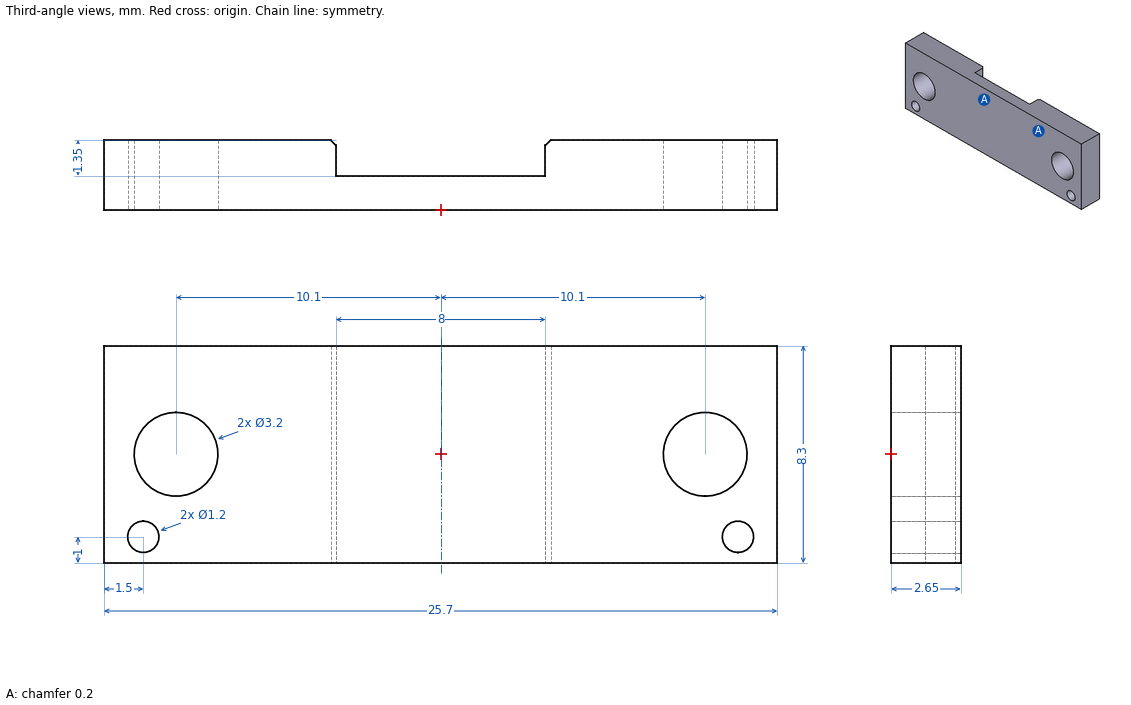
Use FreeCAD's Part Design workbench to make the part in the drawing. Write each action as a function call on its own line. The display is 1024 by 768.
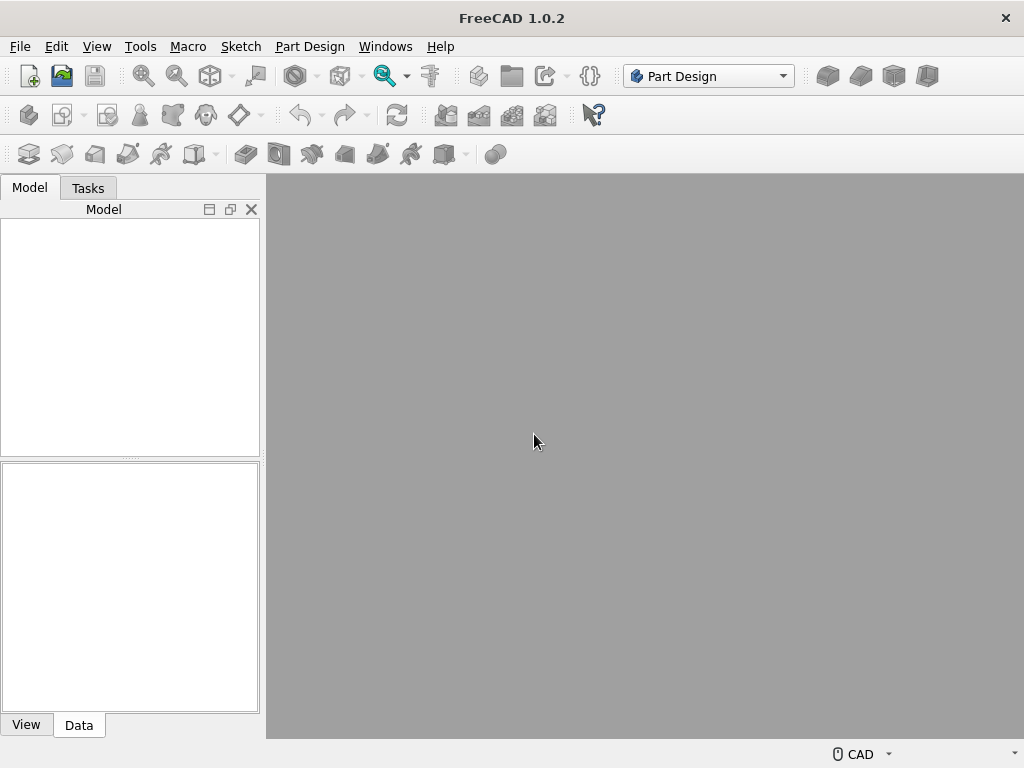
click(29, 76)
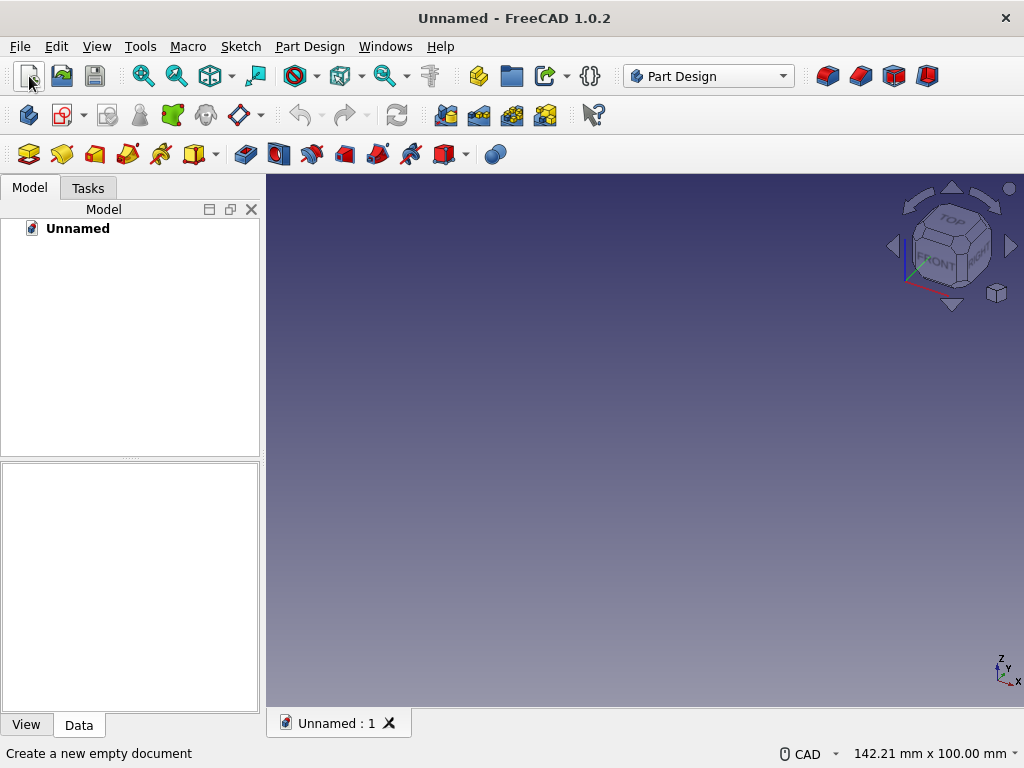
click(62, 116)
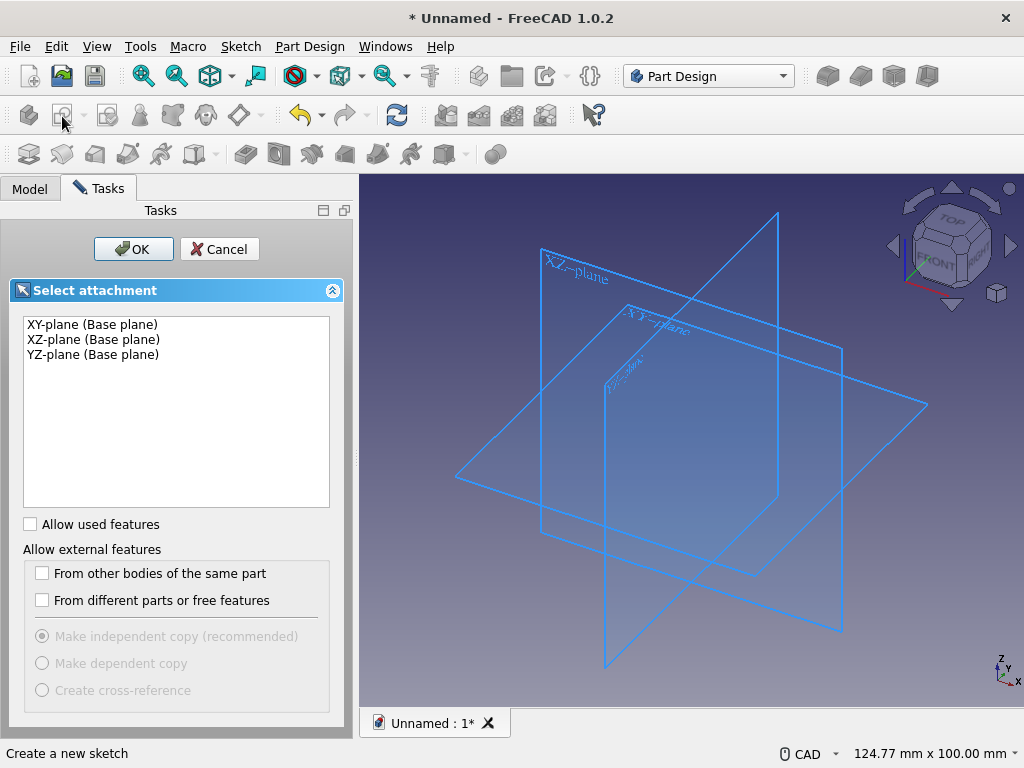
click(84, 340)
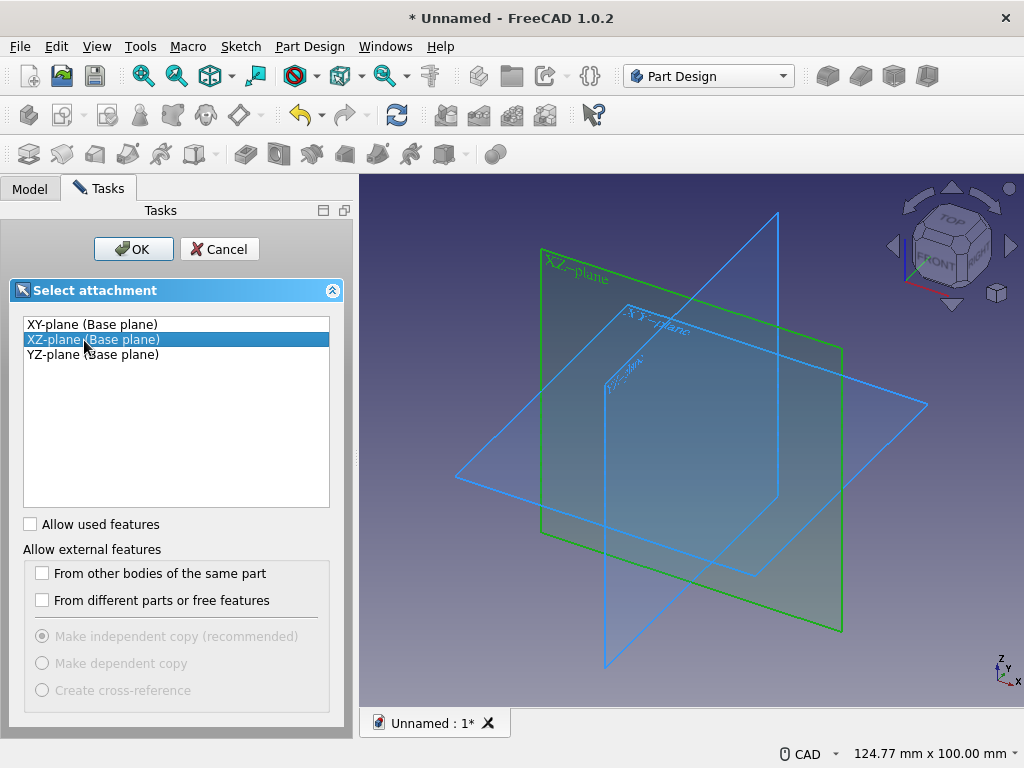
click(134, 249)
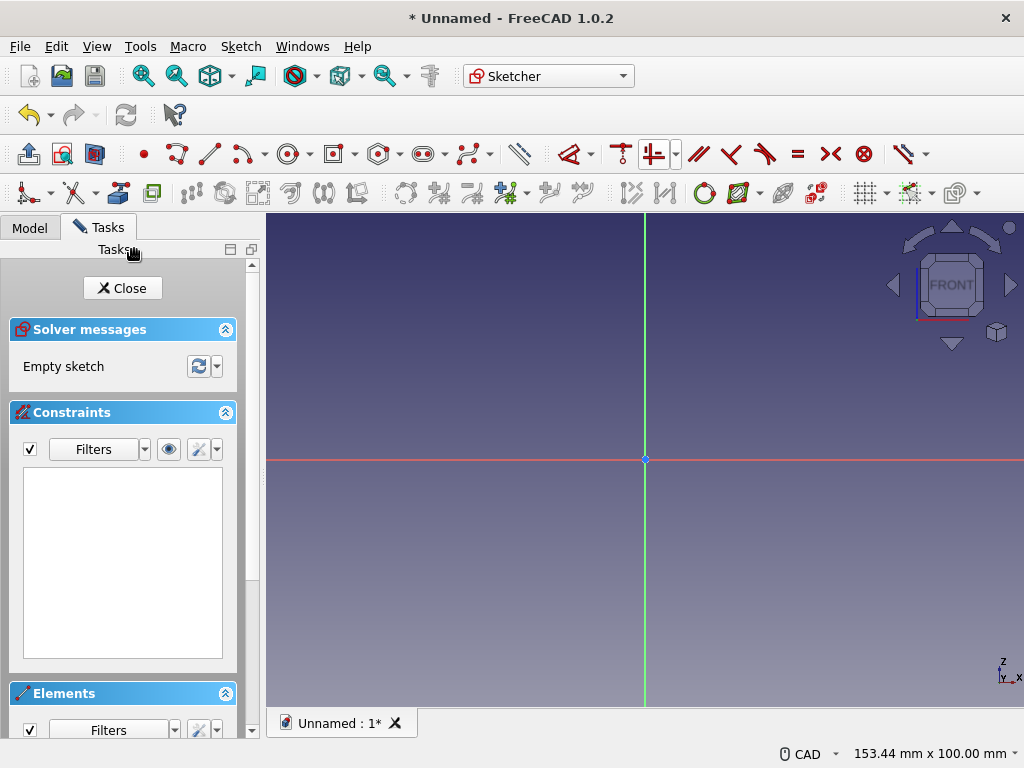
scroll(675, 460, up, 6)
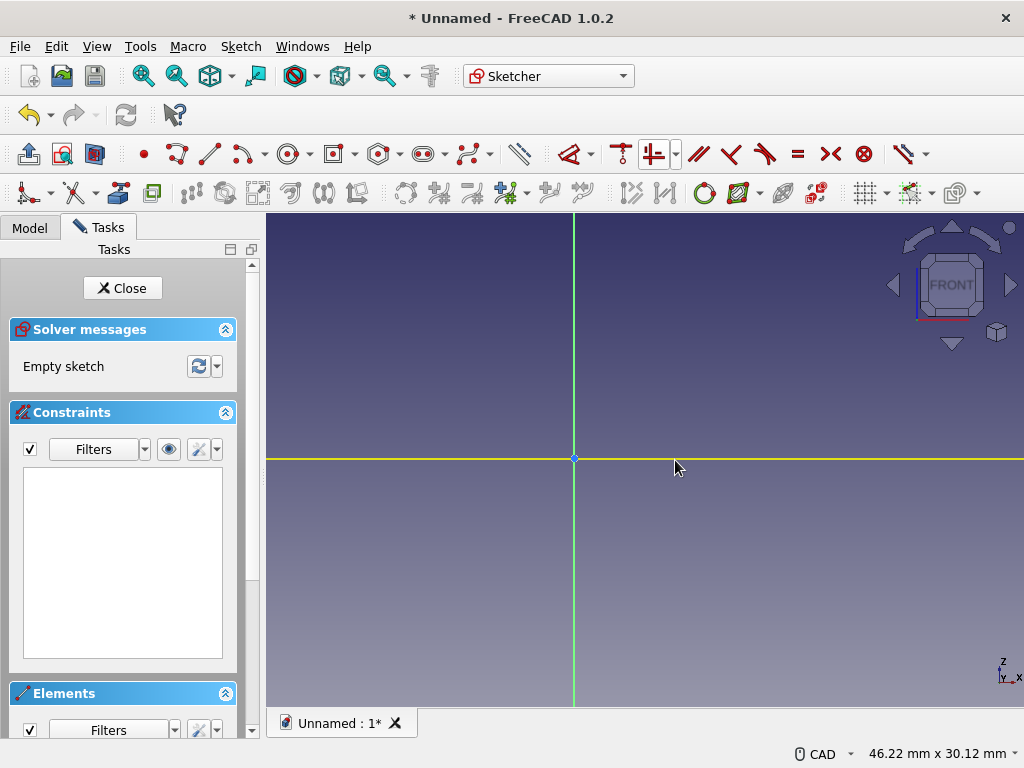
click(332, 154)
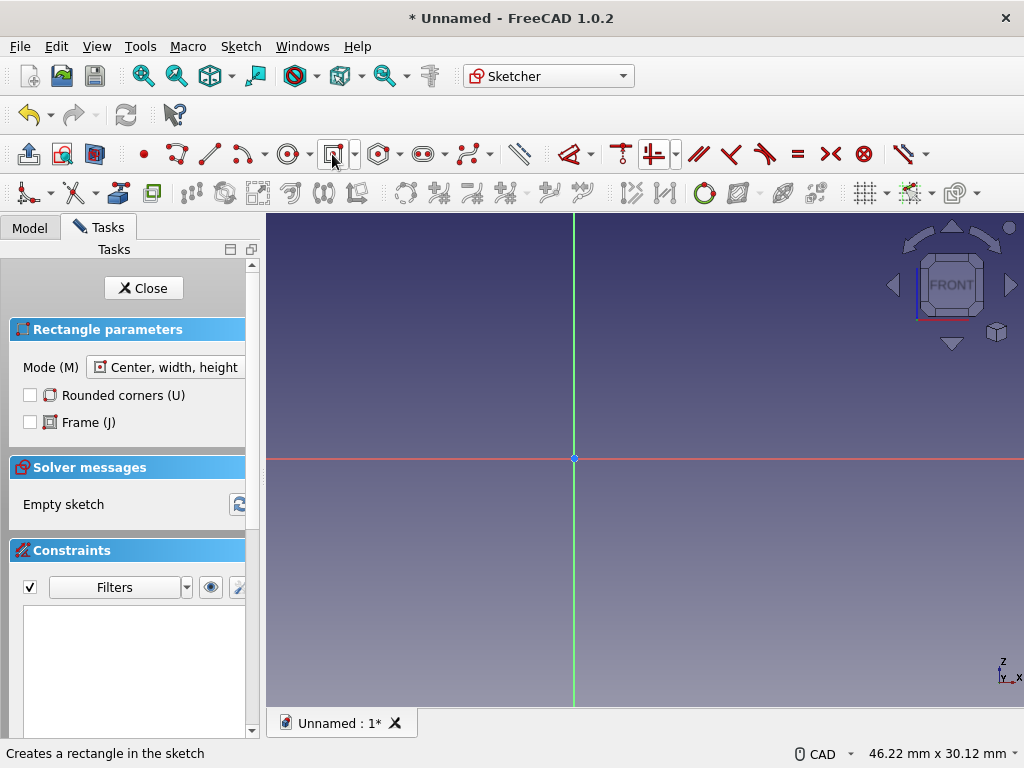
click(574, 459)
move(785, 391)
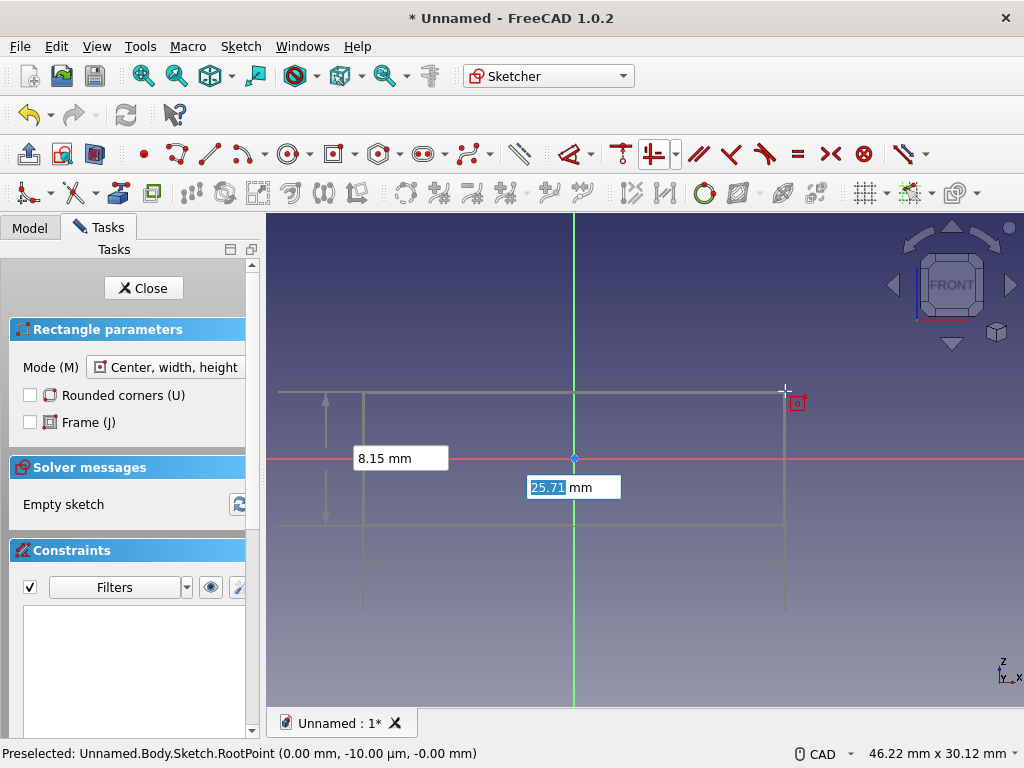
text(25.7)
key(Tab)
text(8.3)
key(Return)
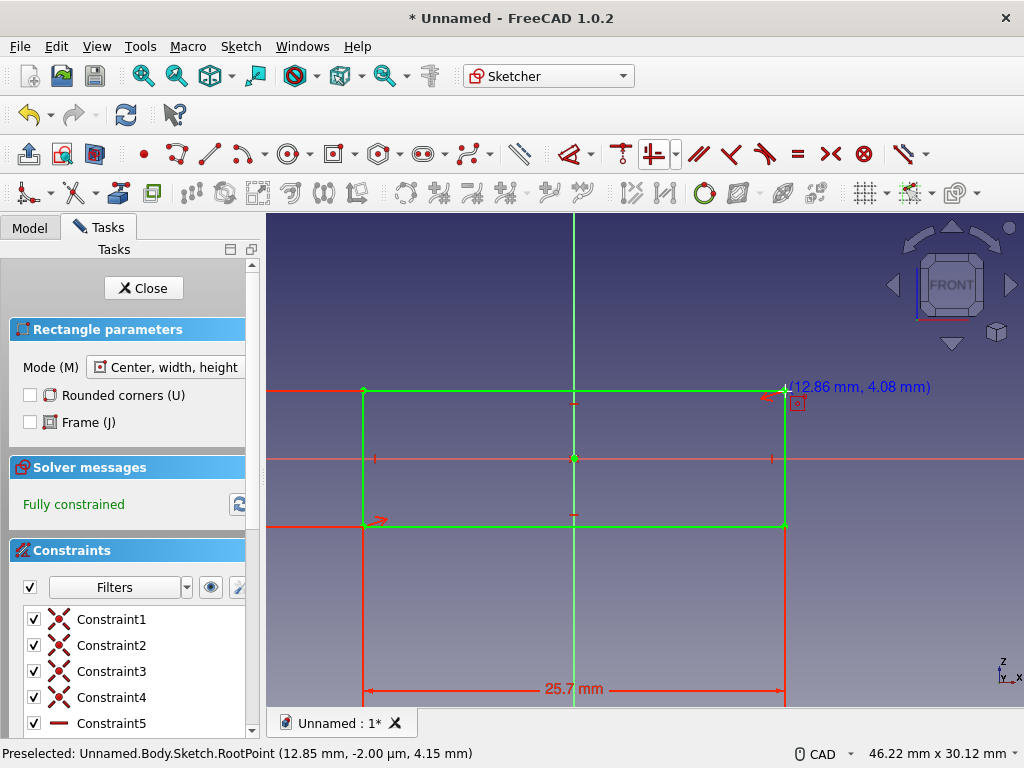
click(288, 154)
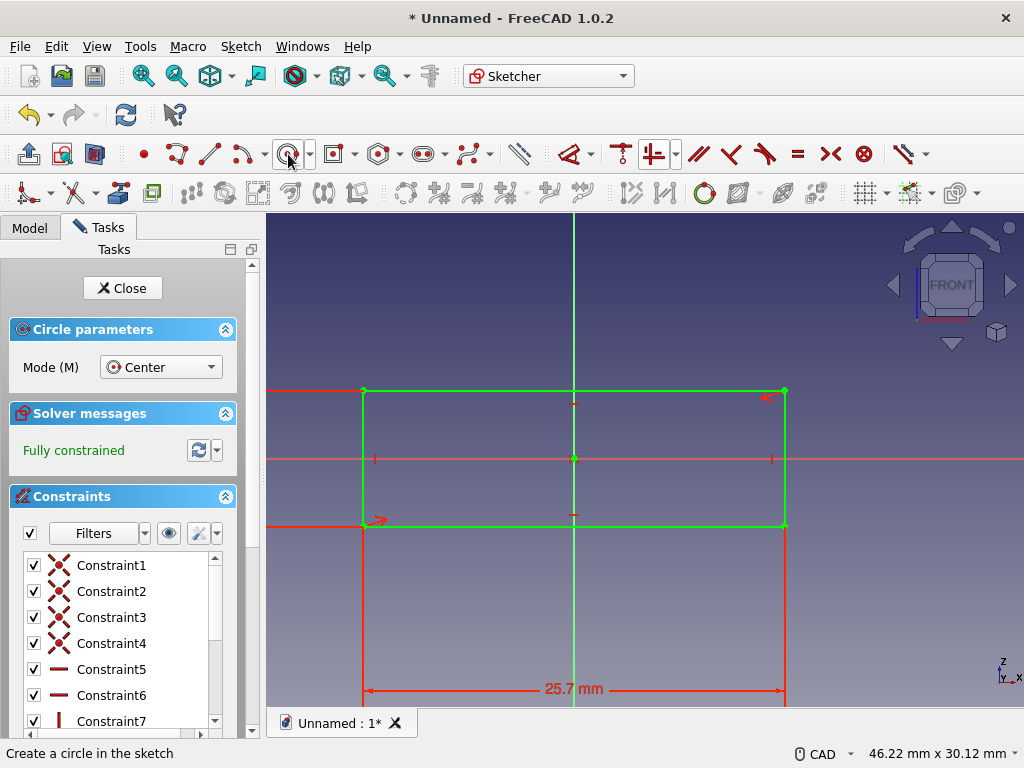
click(408, 459)
move(427, 440)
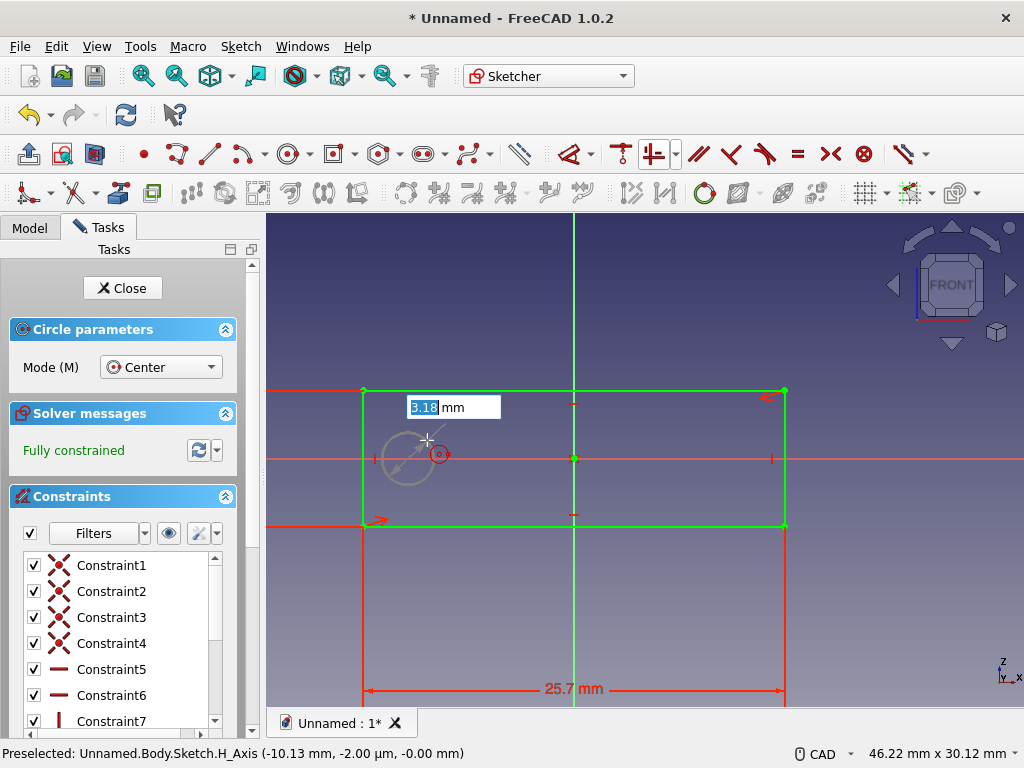
text(3.2)
key(Return)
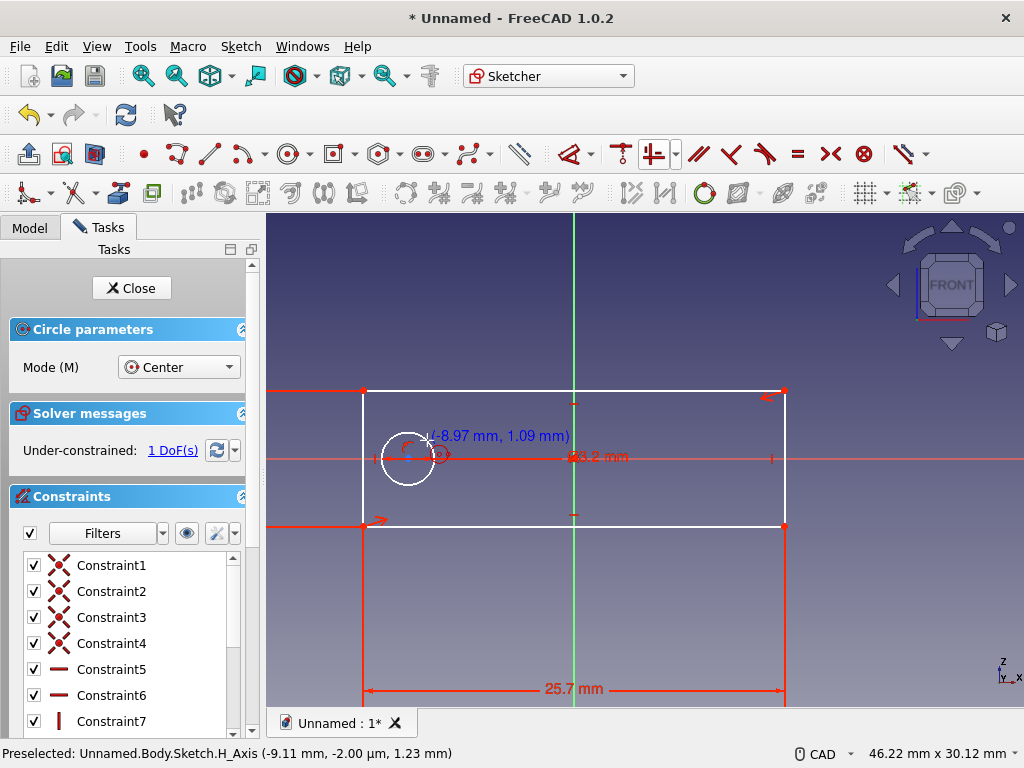
click(740, 459)
move(758, 440)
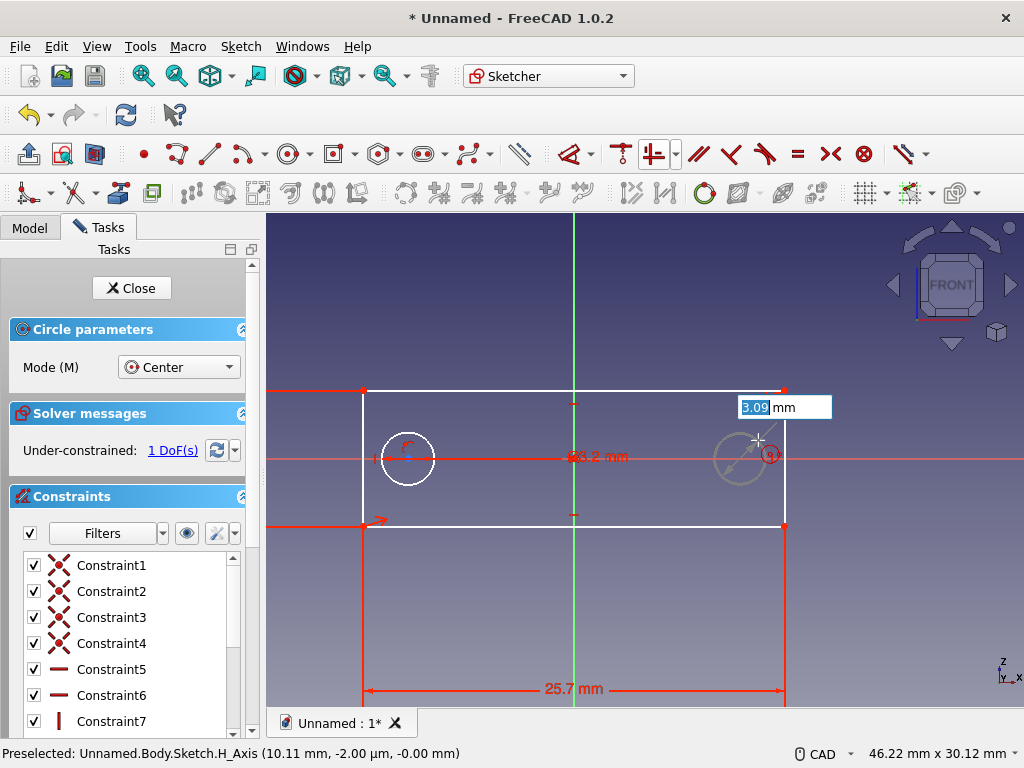
text(3.2)
key(Return)